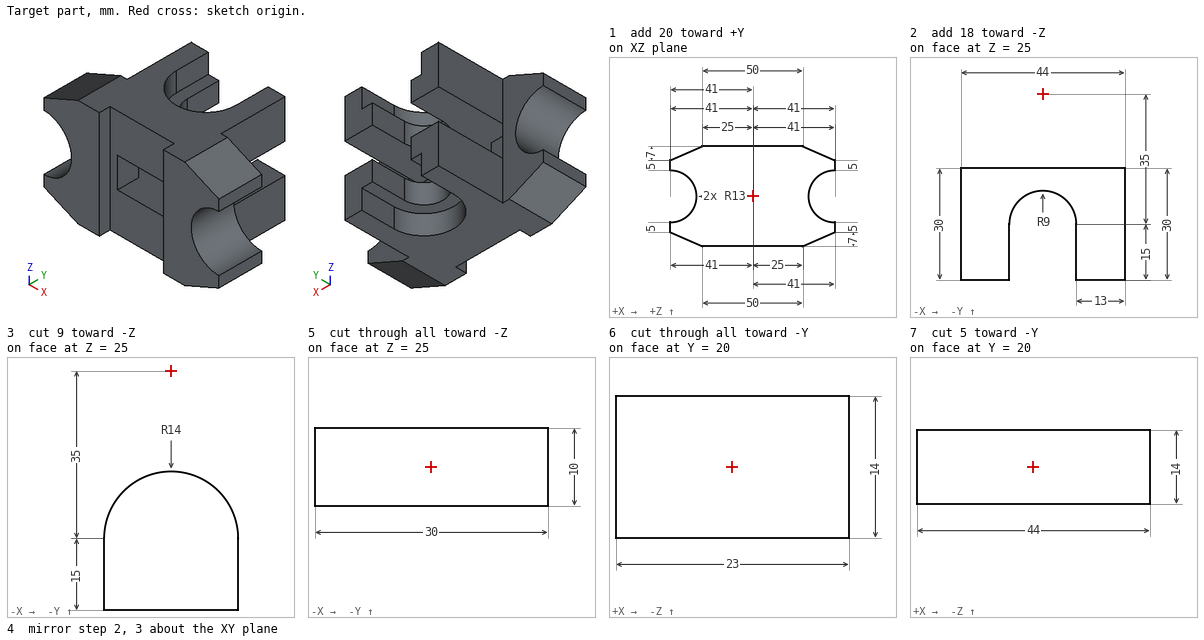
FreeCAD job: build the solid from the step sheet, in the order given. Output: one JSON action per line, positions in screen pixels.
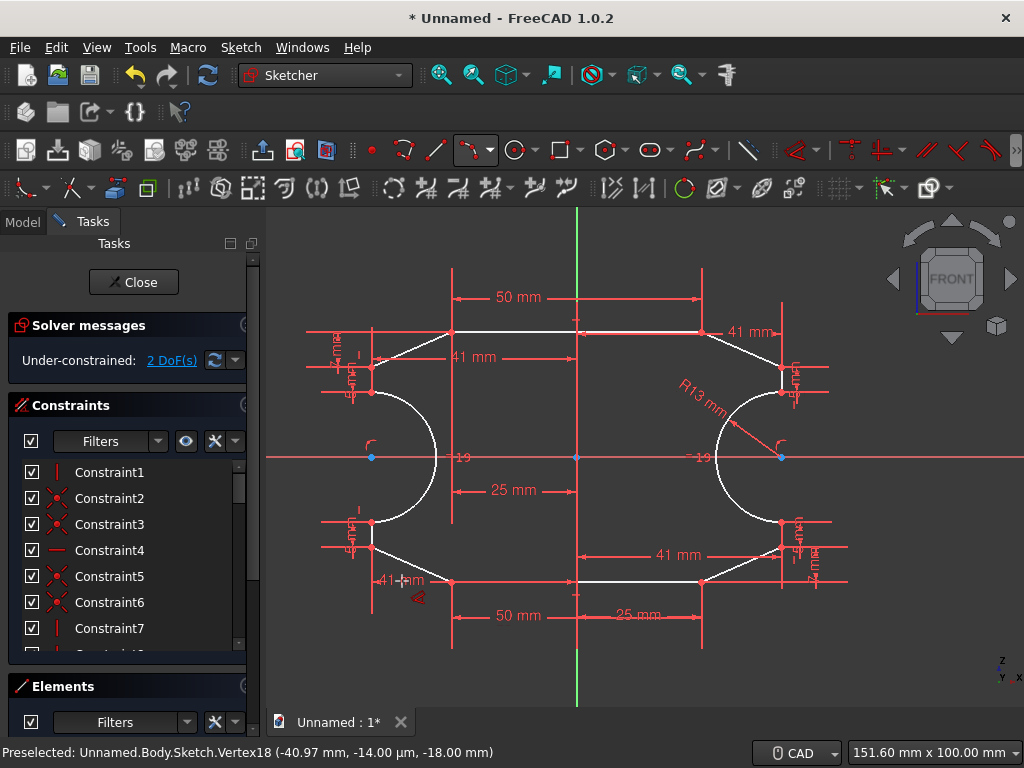
{"action": "left_click", "coordinate": [781, 457]}
{"action": "left_click", "coordinate": [679, 491]}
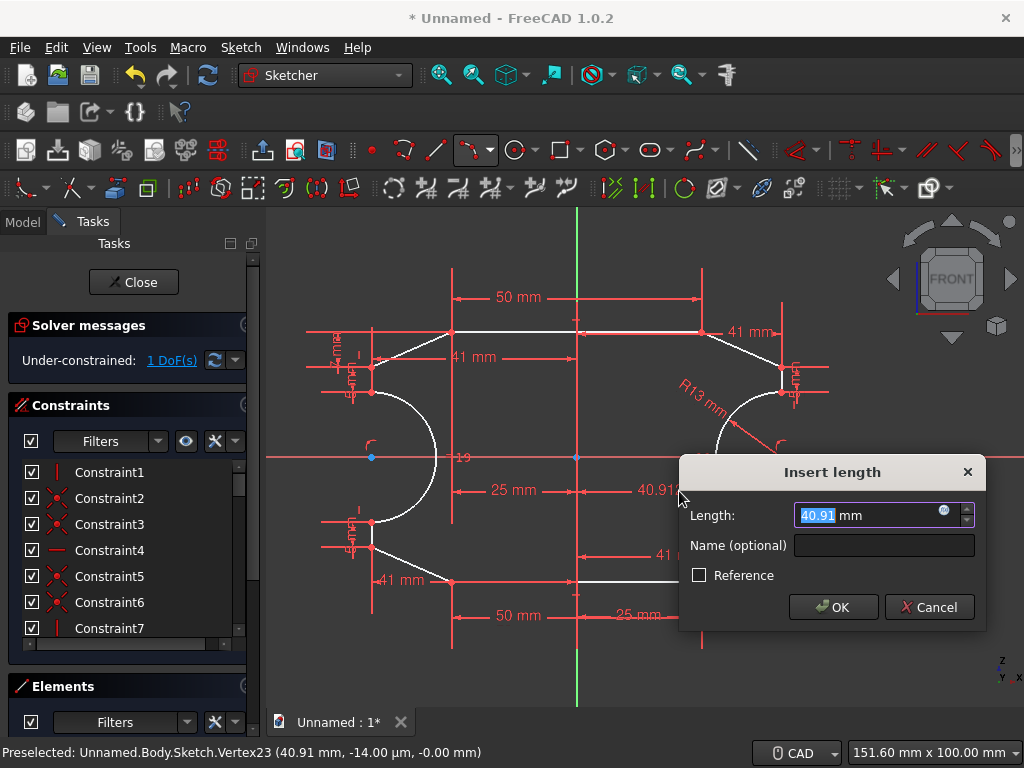
{"action": "type", "text": "41"}
{"action": "key", "text": "Return"}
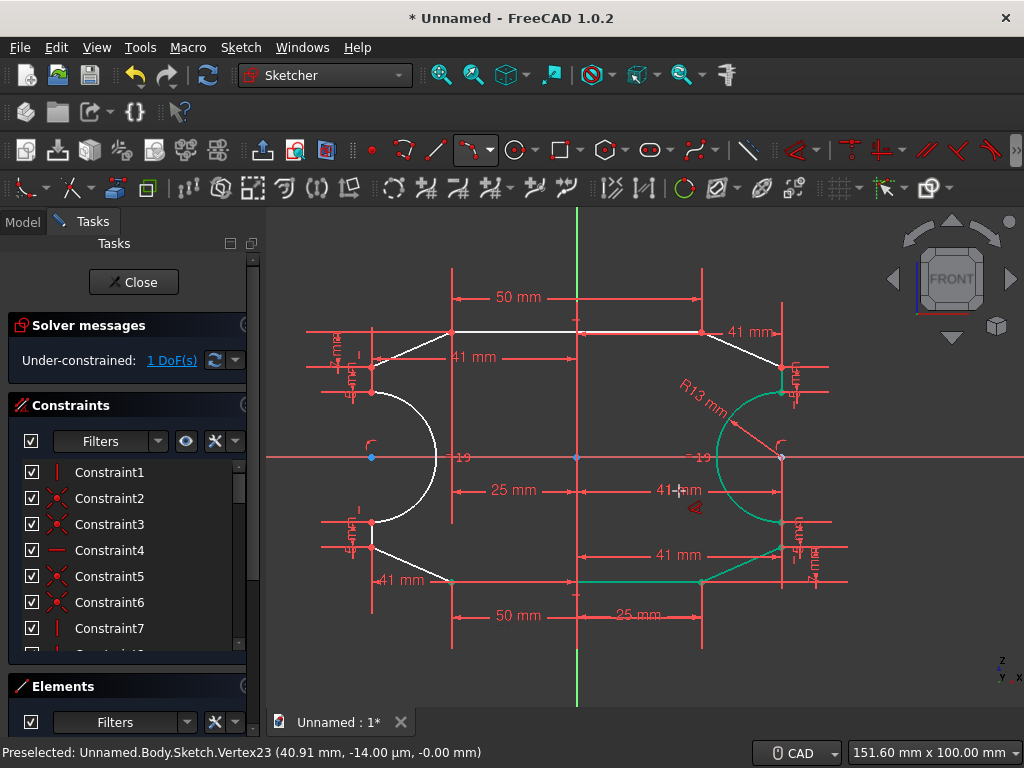
{"action": "left_click", "coordinate": [371, 457]}
{"action": "left_click", "coordinate": [402, 491]}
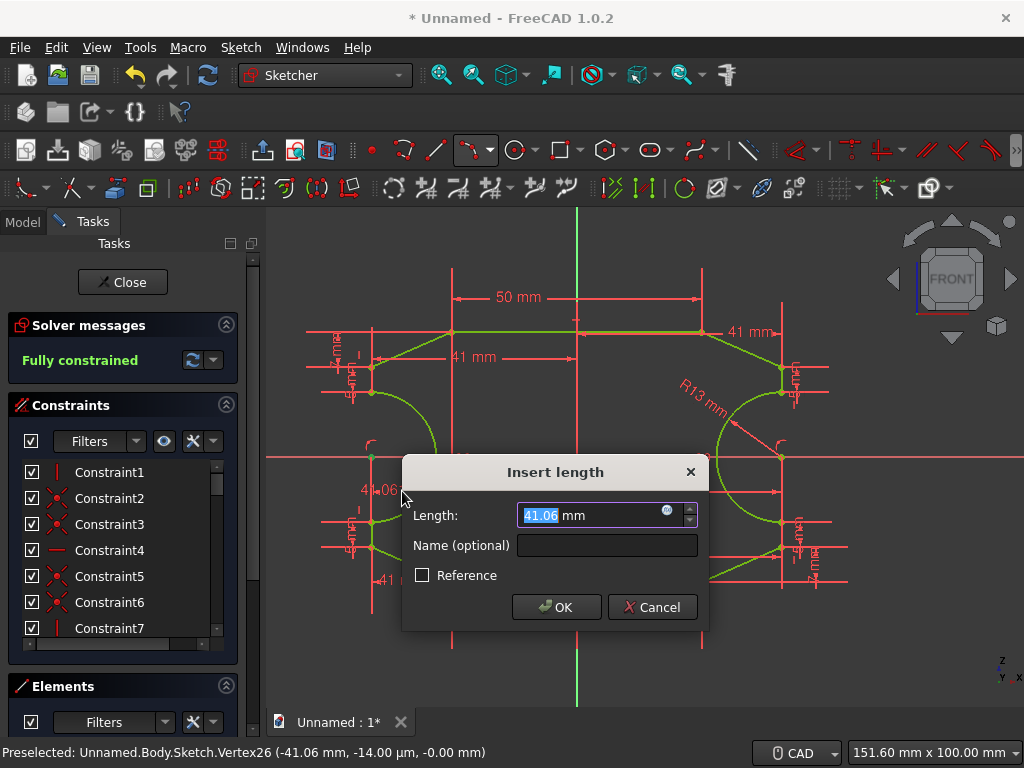
{"action": "type", "text": "41"}
{"action": "key", "text": "Return"}
{"action": "key", "text": "Escape"}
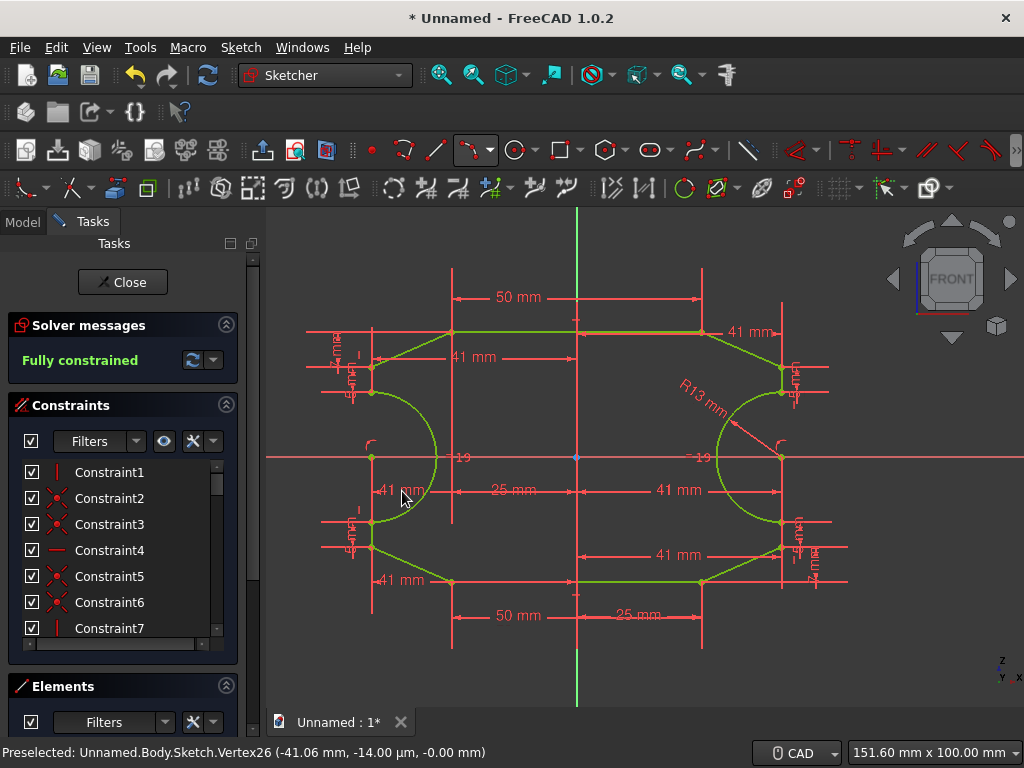
{"action": "left_click", "coordinate": [123, 282]}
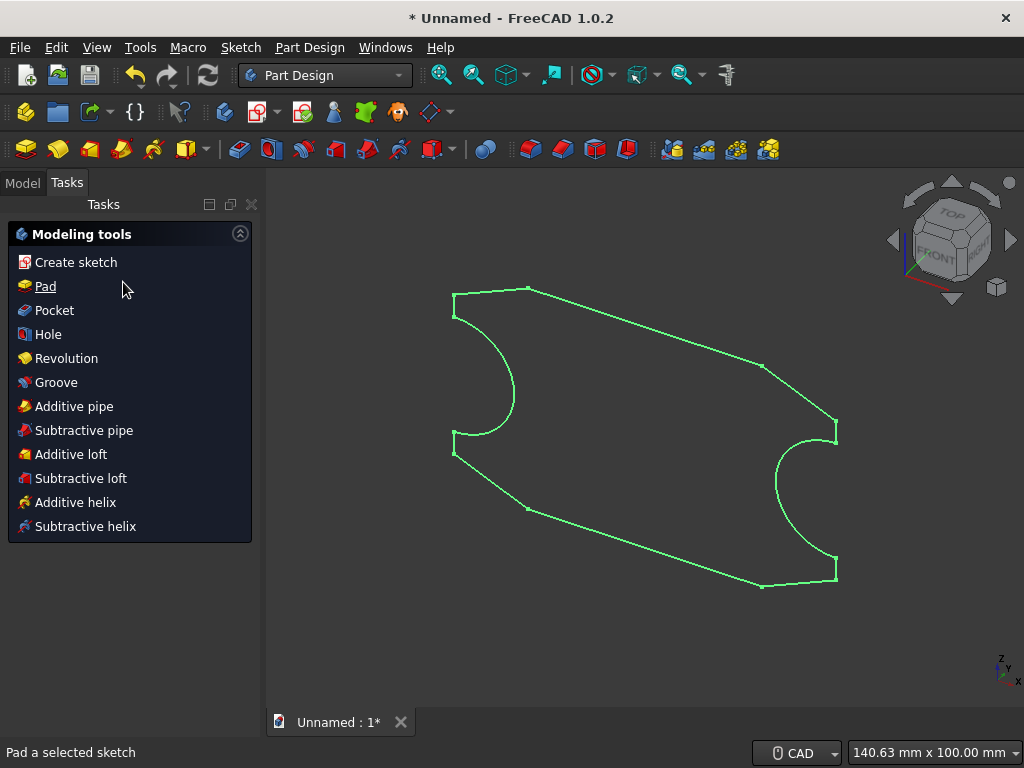
{"action": "left_click", "coordinate": [26, 150]}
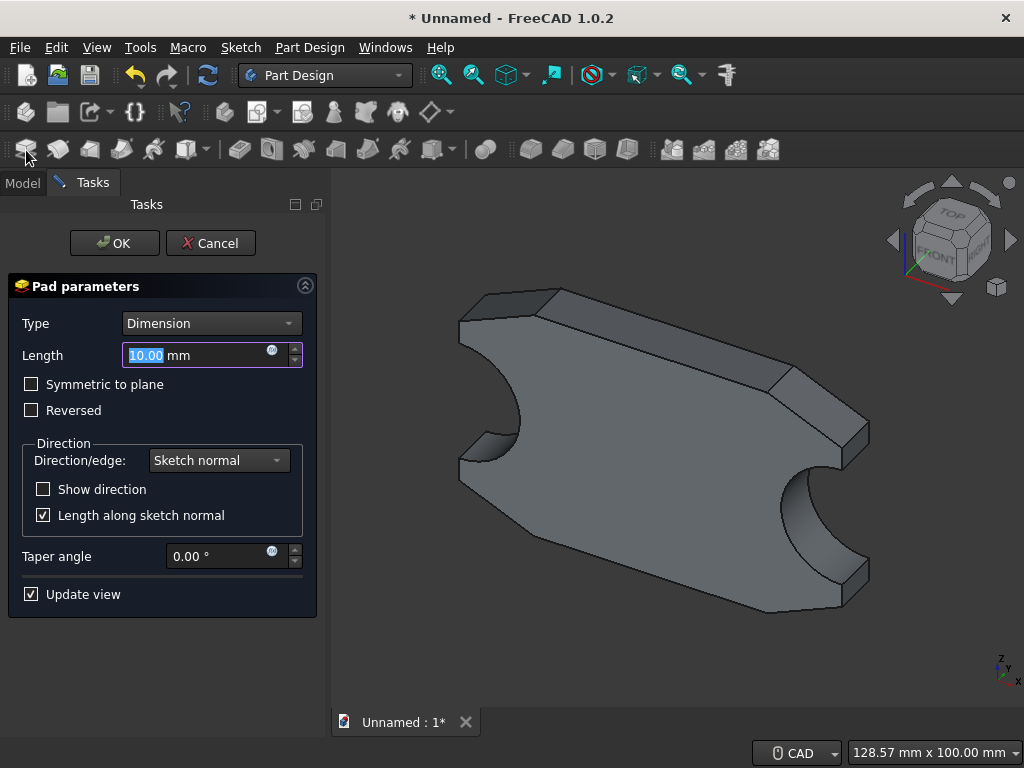
{"action": "type", "text": "20"}
{"action": "key", "text": "Tab"}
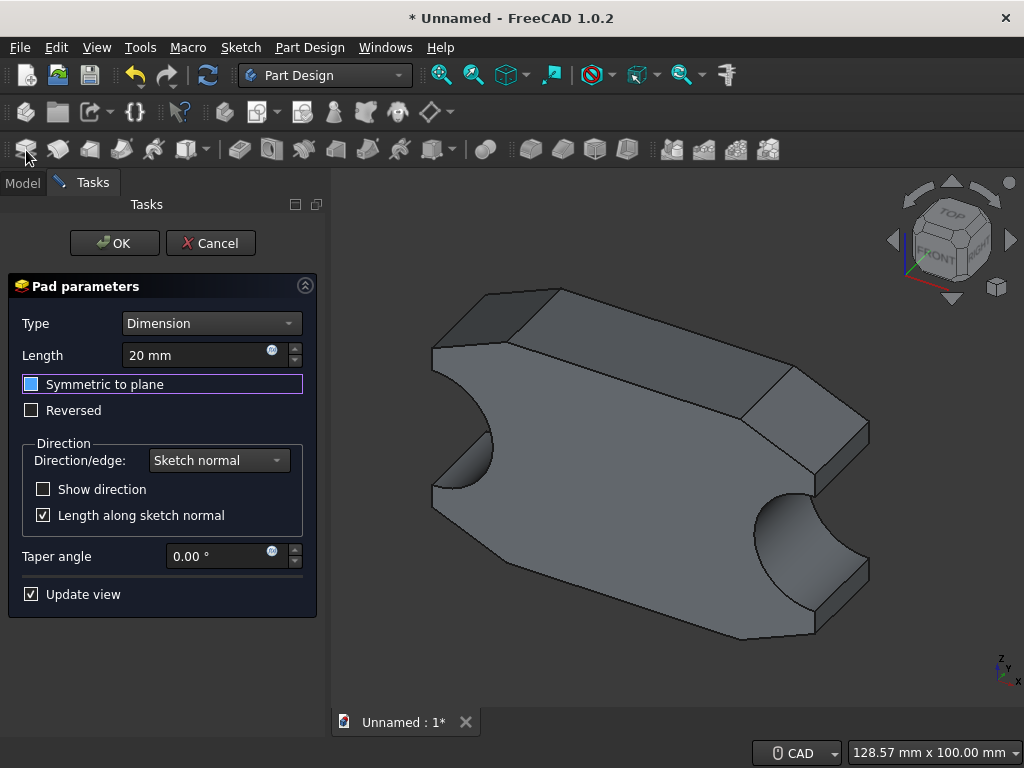
{"action": "left_click", "coordinate": [30, 410]}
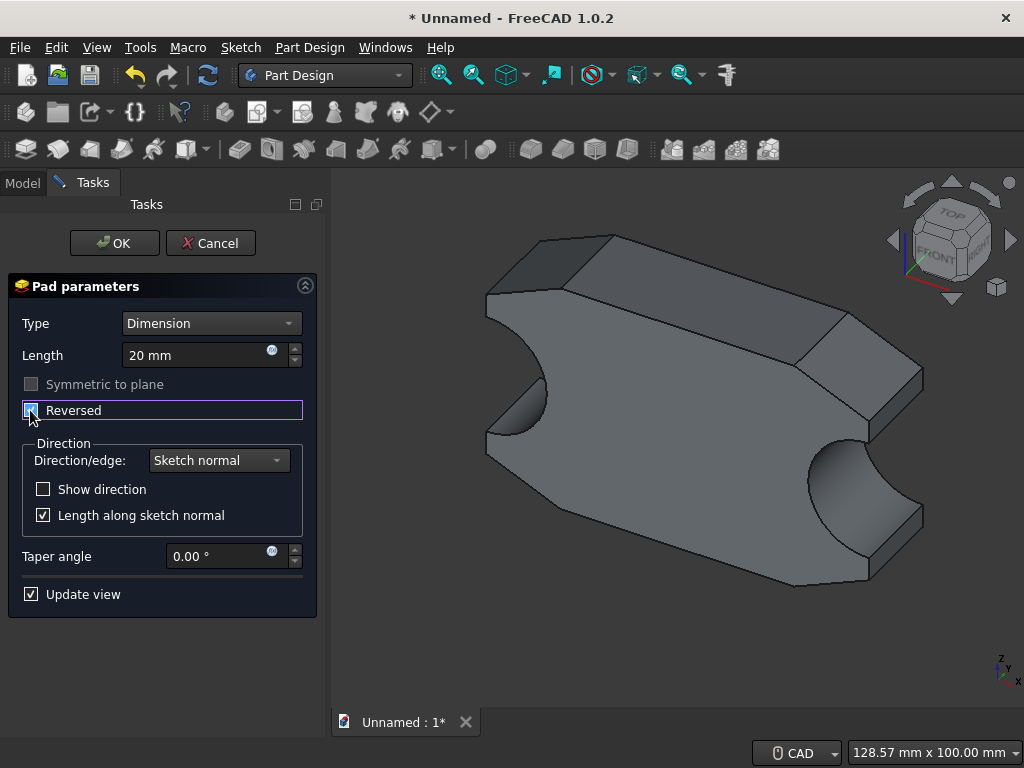
{"action": "left_click", "coordinate": [115, 243]}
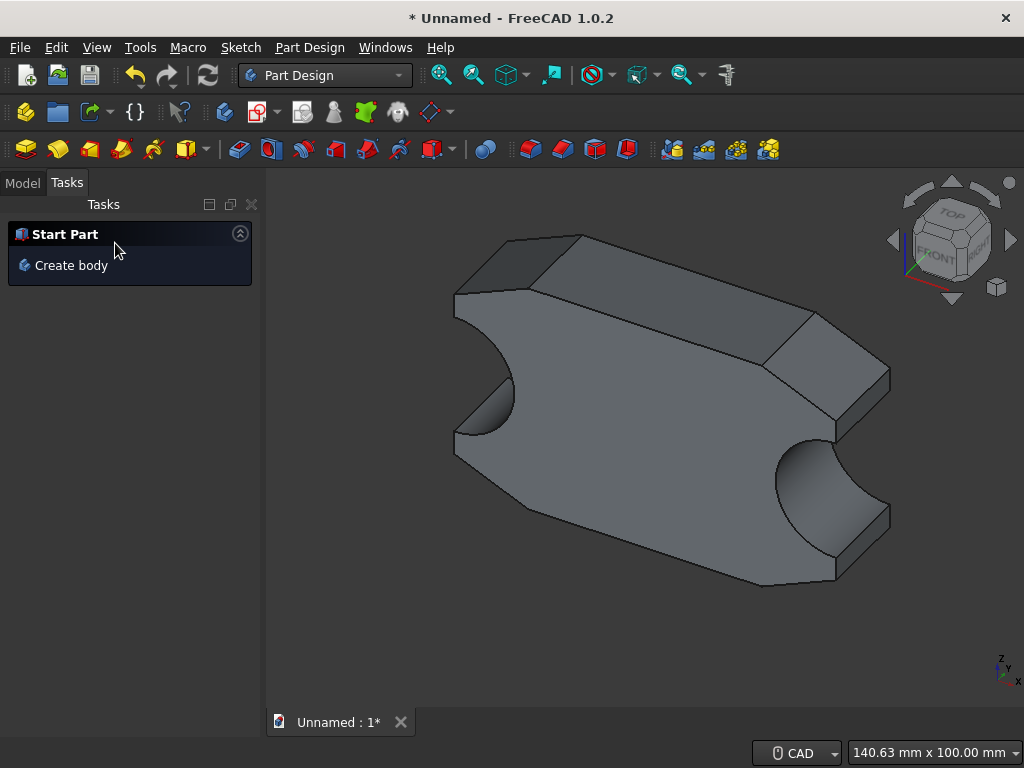
{"action": "left_click", "coordinate": [739, 321]}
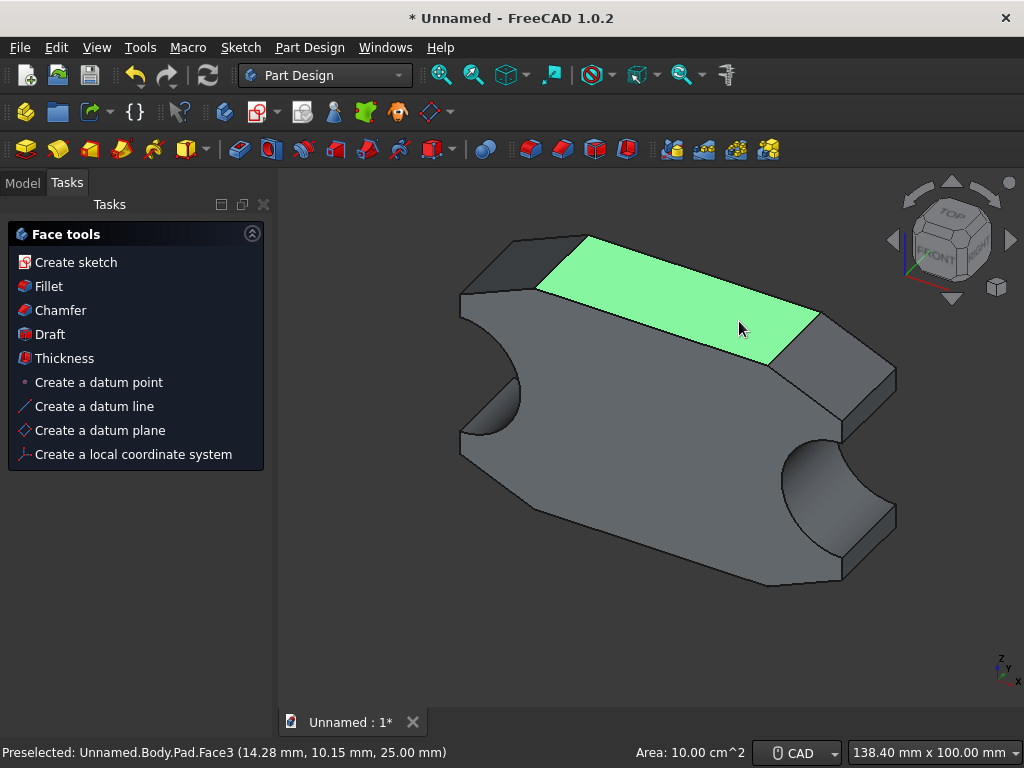
{"action": "left_click", "coordinate": [258, 112]}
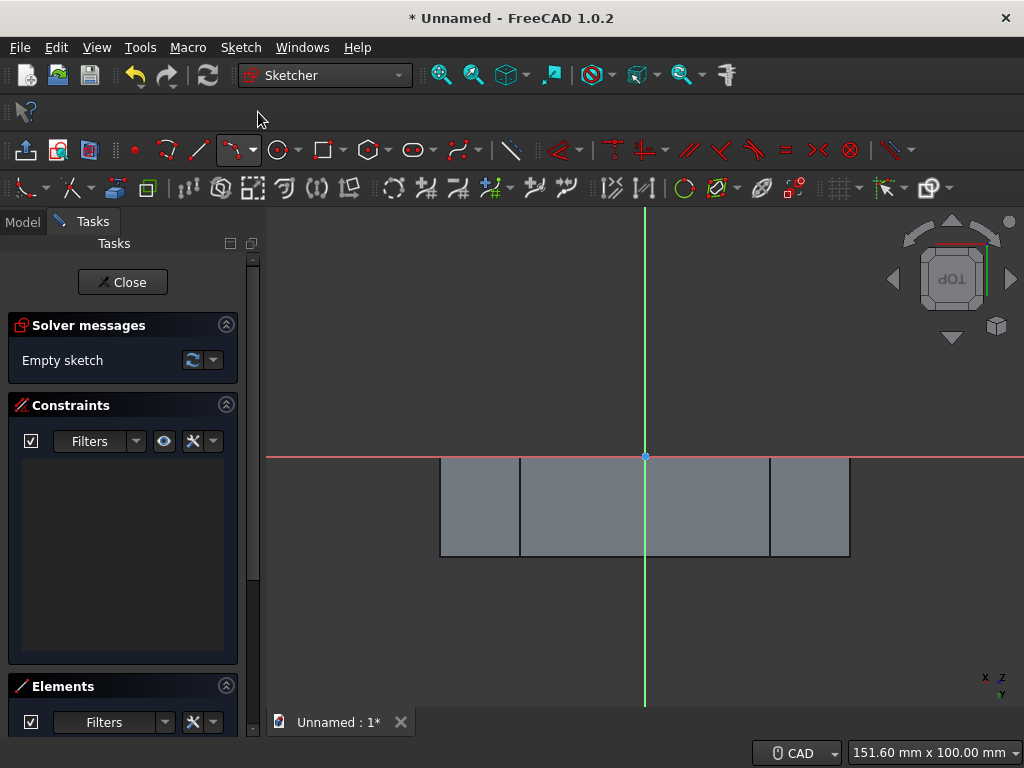
{"action": "scroll", "coordinate": [294, 235], "scroll_direction": "down", "scroll_amount": 1}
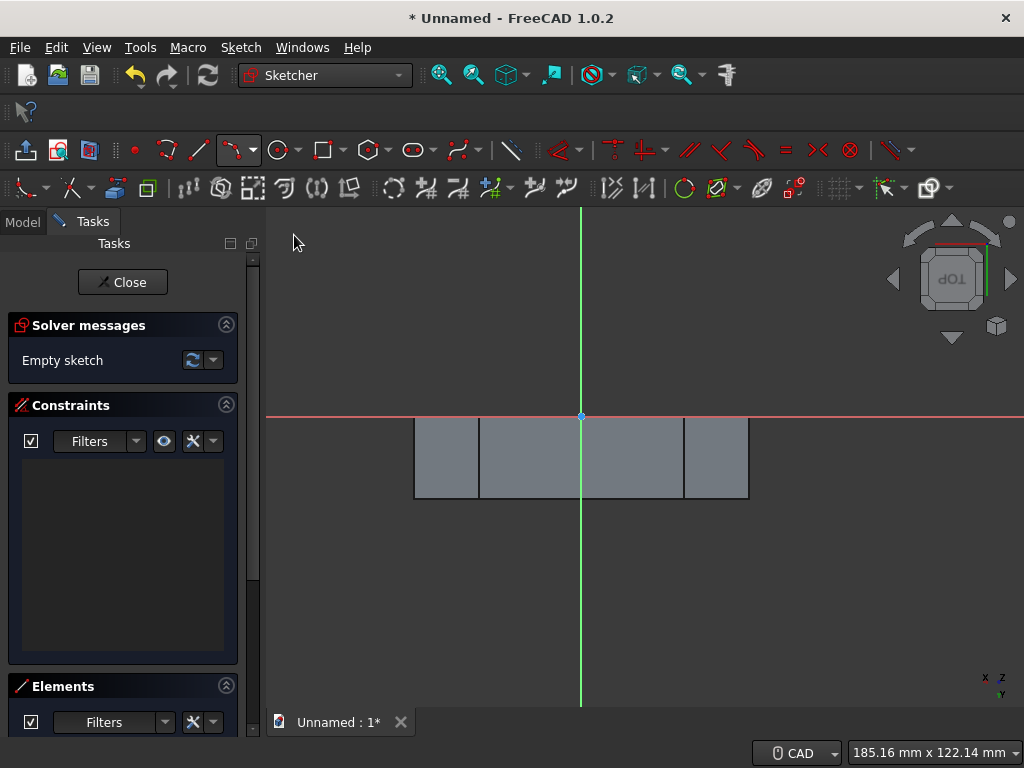
{"action": "scroll", "coordinate": [591, 645], "scroll_direction": "up", "scroll_amount": 2}